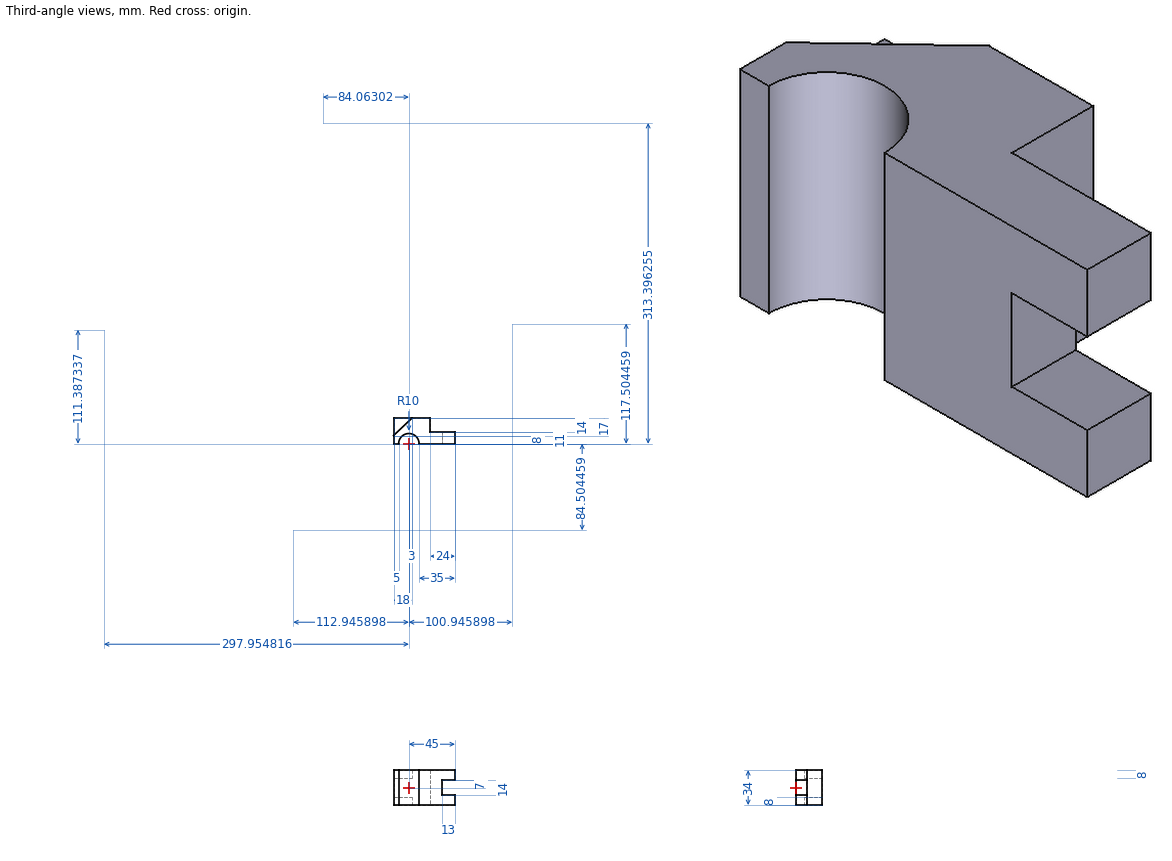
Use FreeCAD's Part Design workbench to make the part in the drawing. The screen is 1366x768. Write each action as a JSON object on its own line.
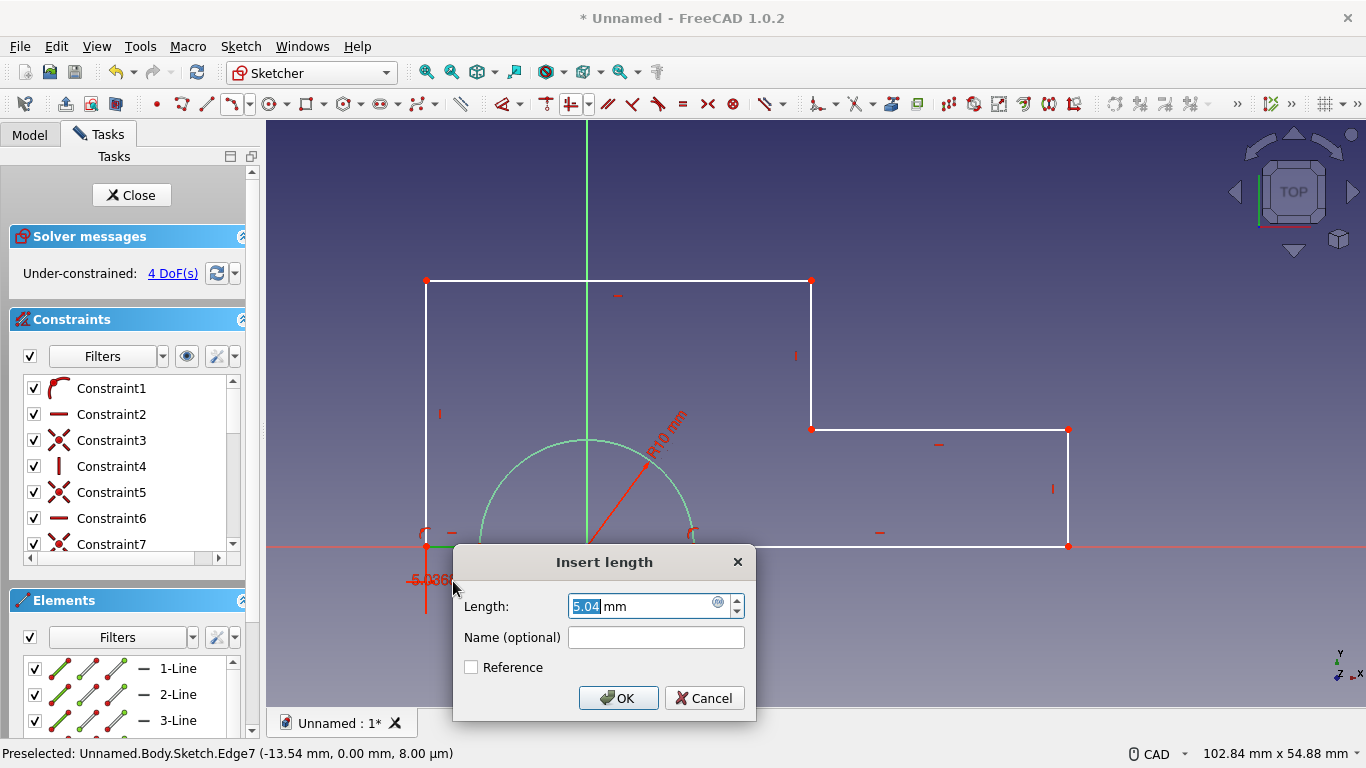
{"action": "type", "text": "5"}
{"action": "key", "text": "Return"}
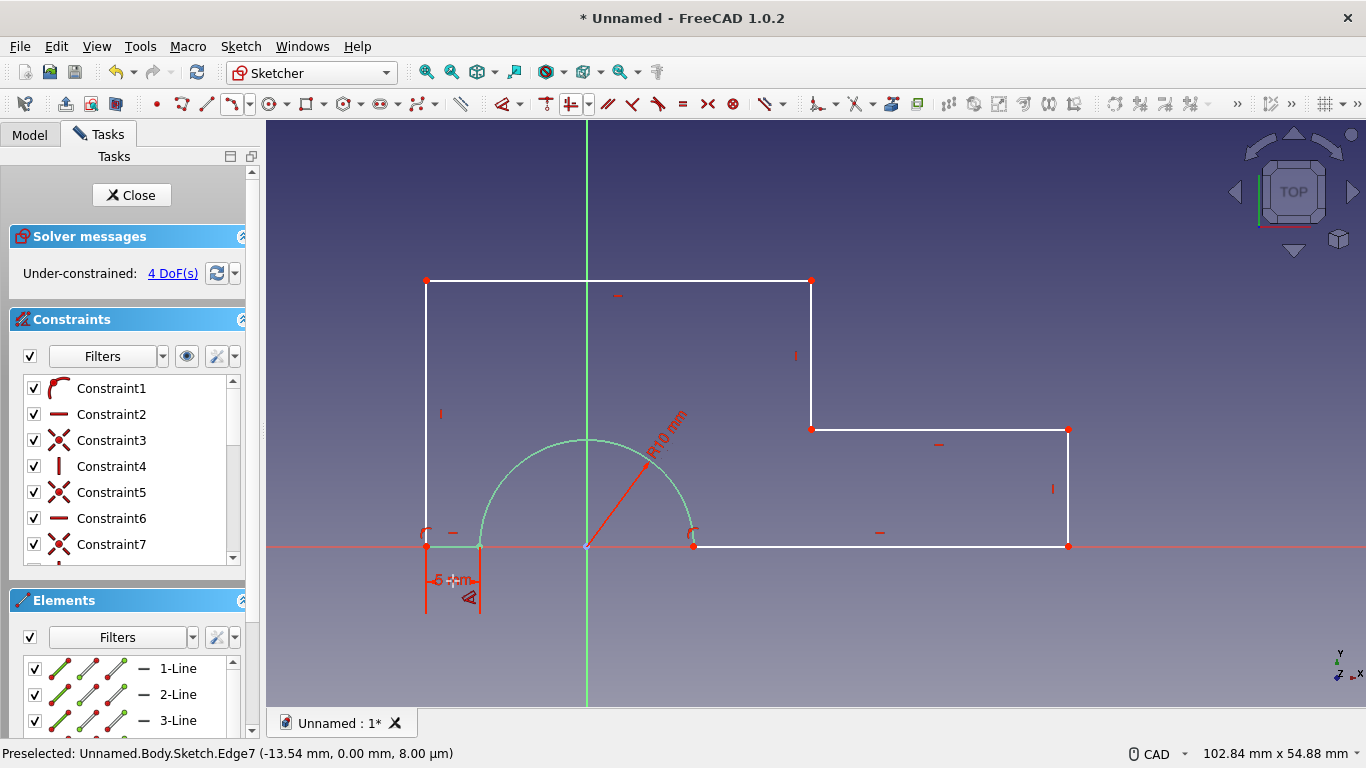
{"action": "left_click", "coordinate": [806, 547]}
{"action": "left_click", "coordinate": [881, 581]}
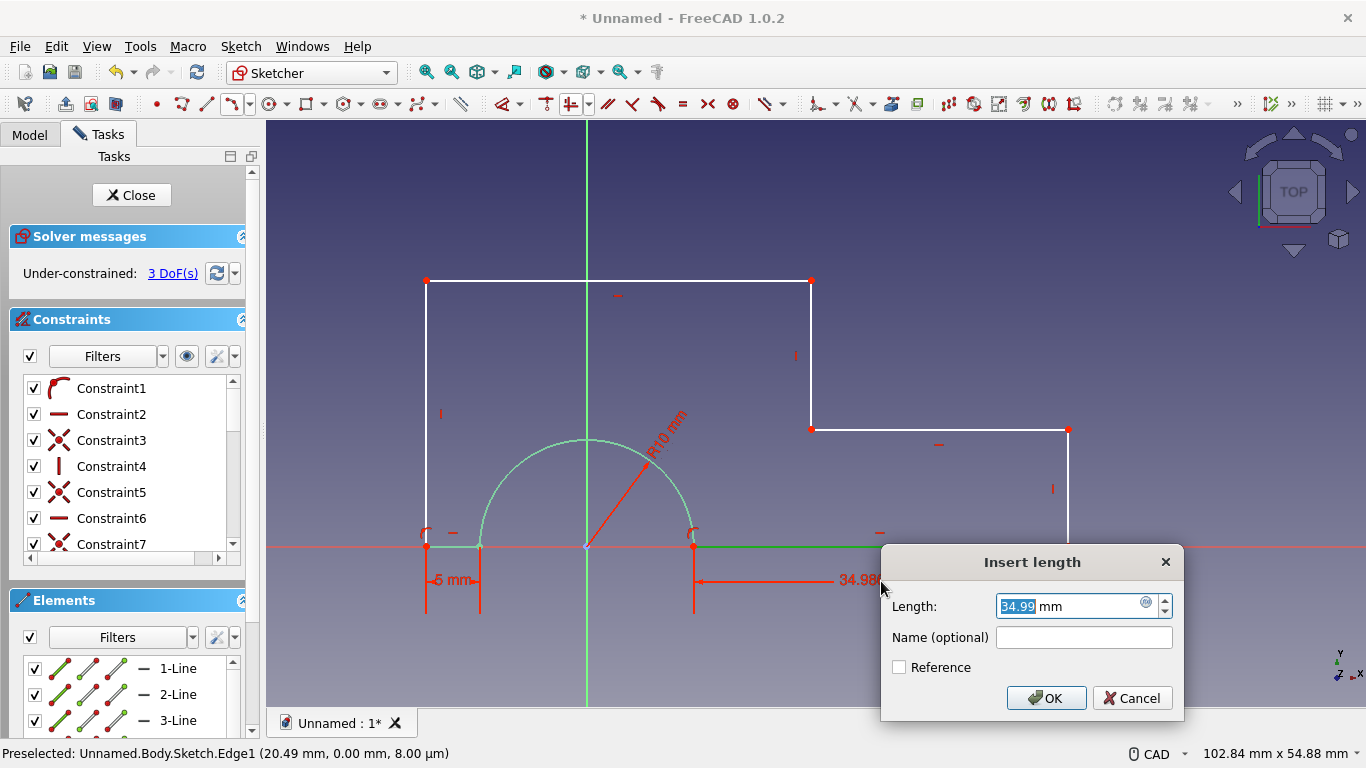
{"action": "type", "text": "35"}
{"action": "key", "text": "Return"}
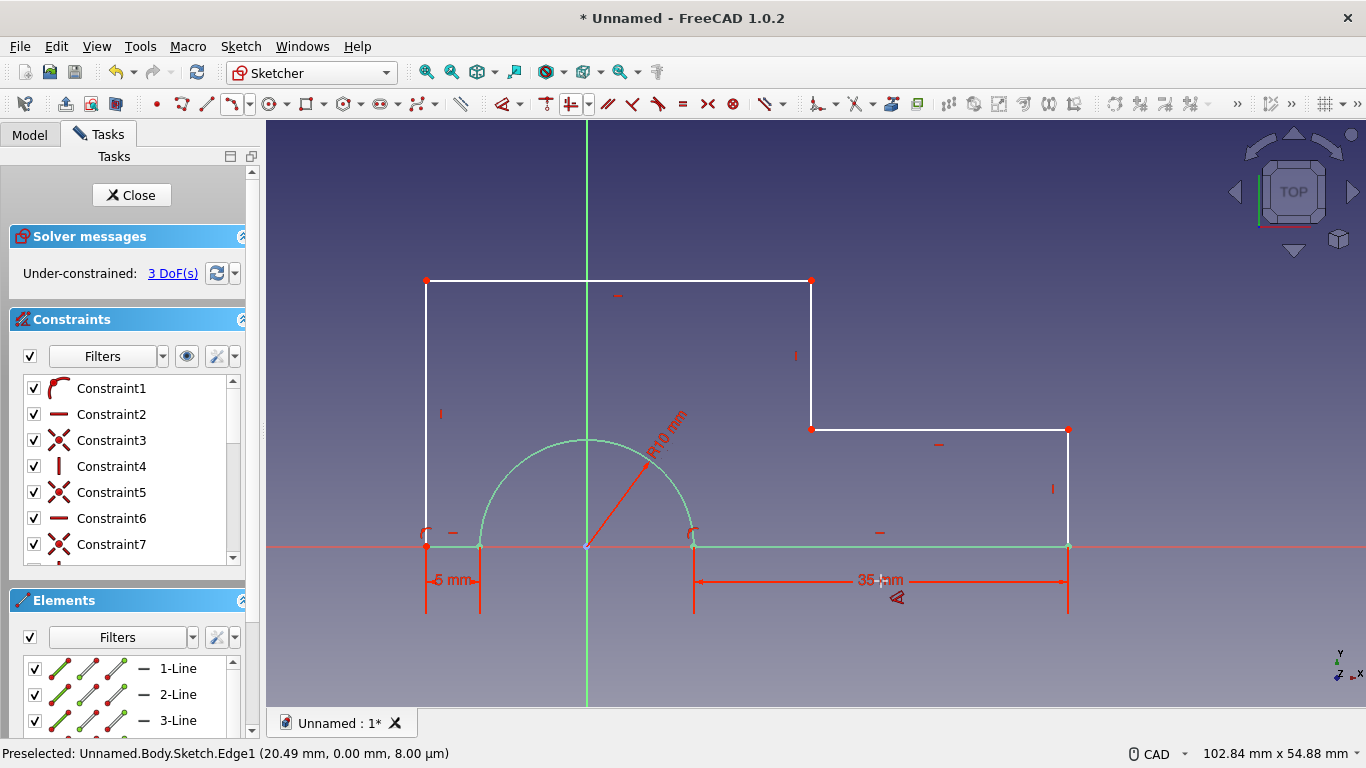
{"action": "left_click", "coordinate": [1068, 512]}
{"action": "left_click", "coordinate": [1102, 488]}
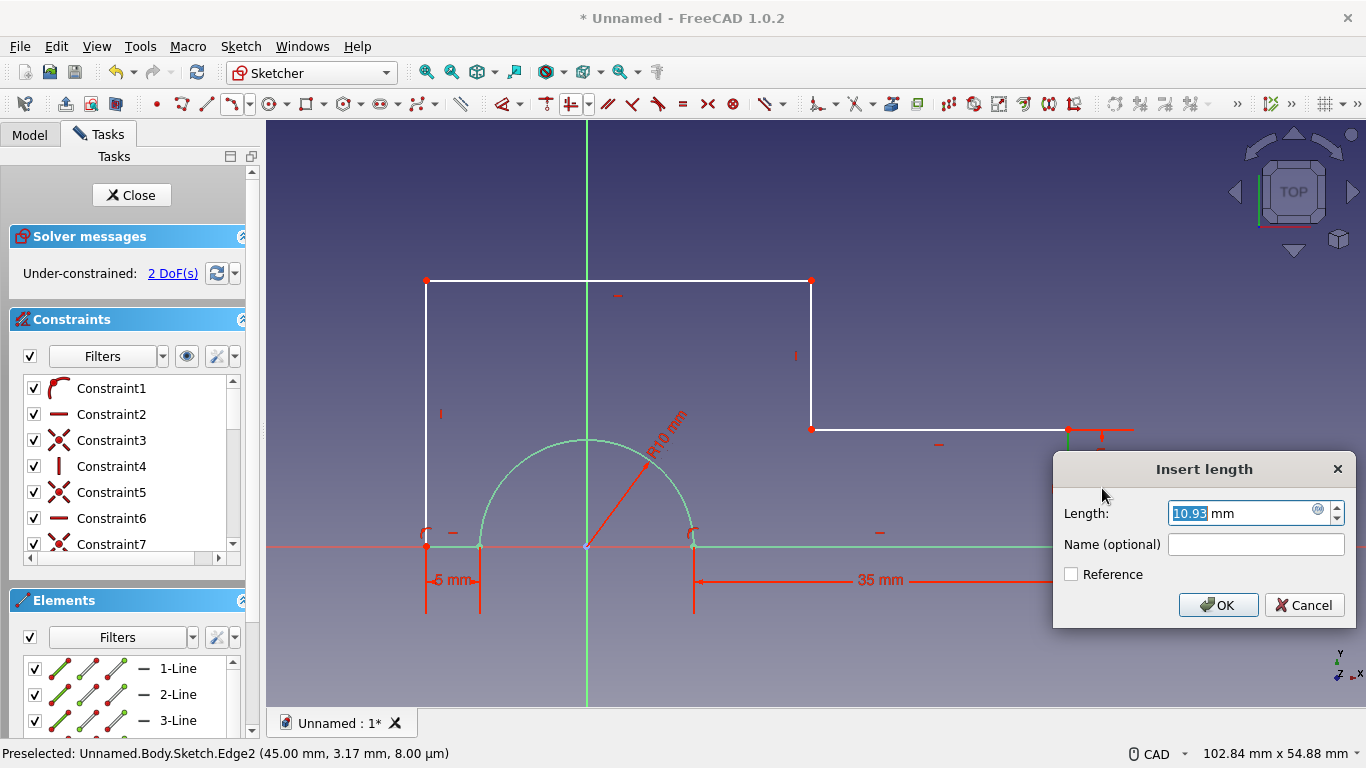
{"action": "type", "text": "11"}
{"action": "key", "text": "Return"}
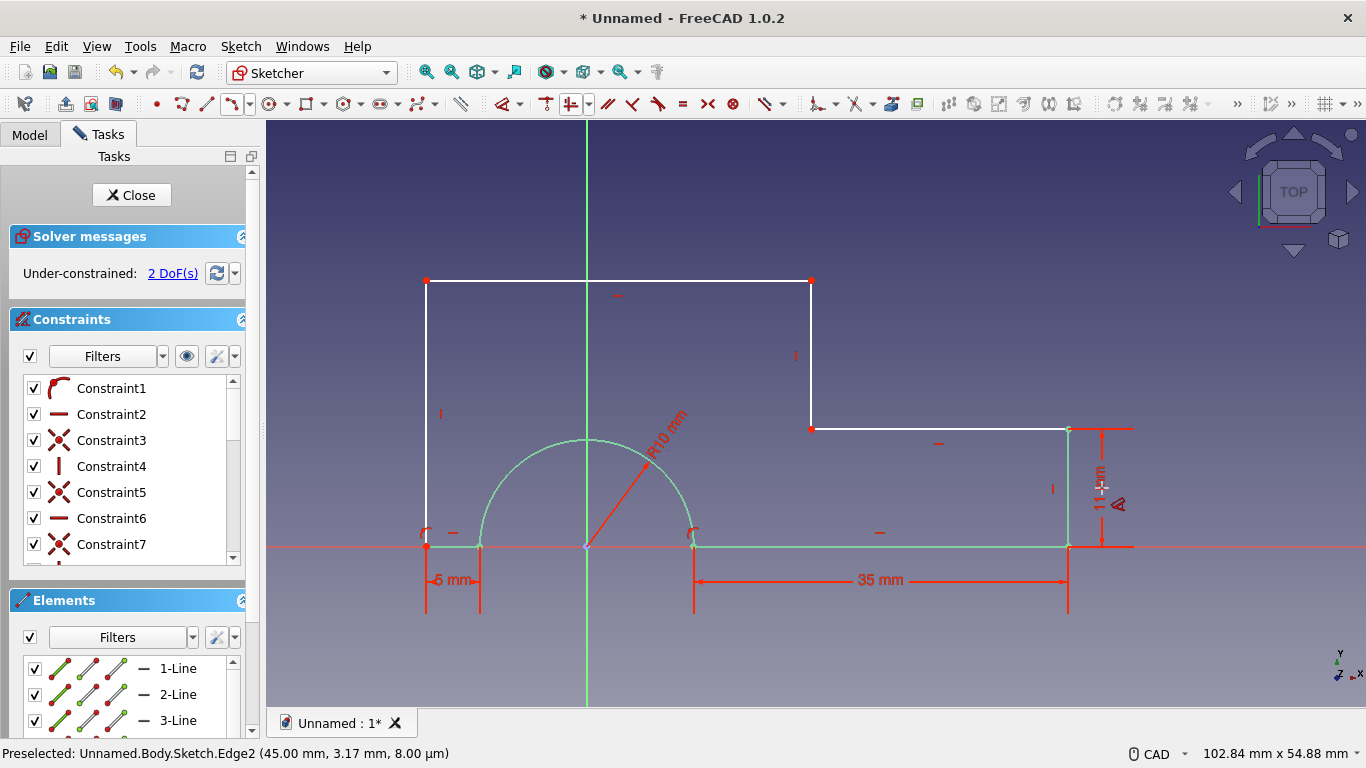
{"action": "left_click", "coordinate": [991, 429]}
{"action": "left_click", "coordinate": [940, 463]}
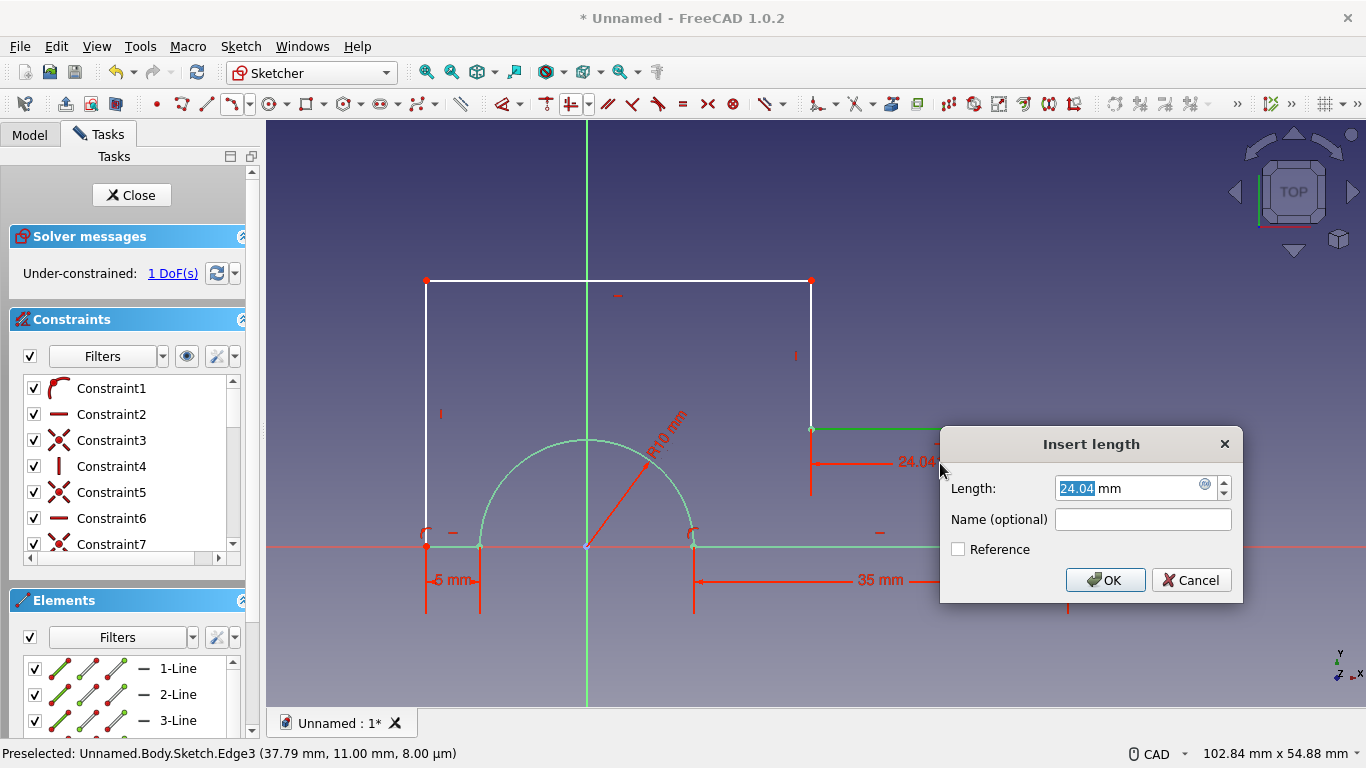
{"action": "type", "text": "24"}
{"action": "key", "text": "Return"}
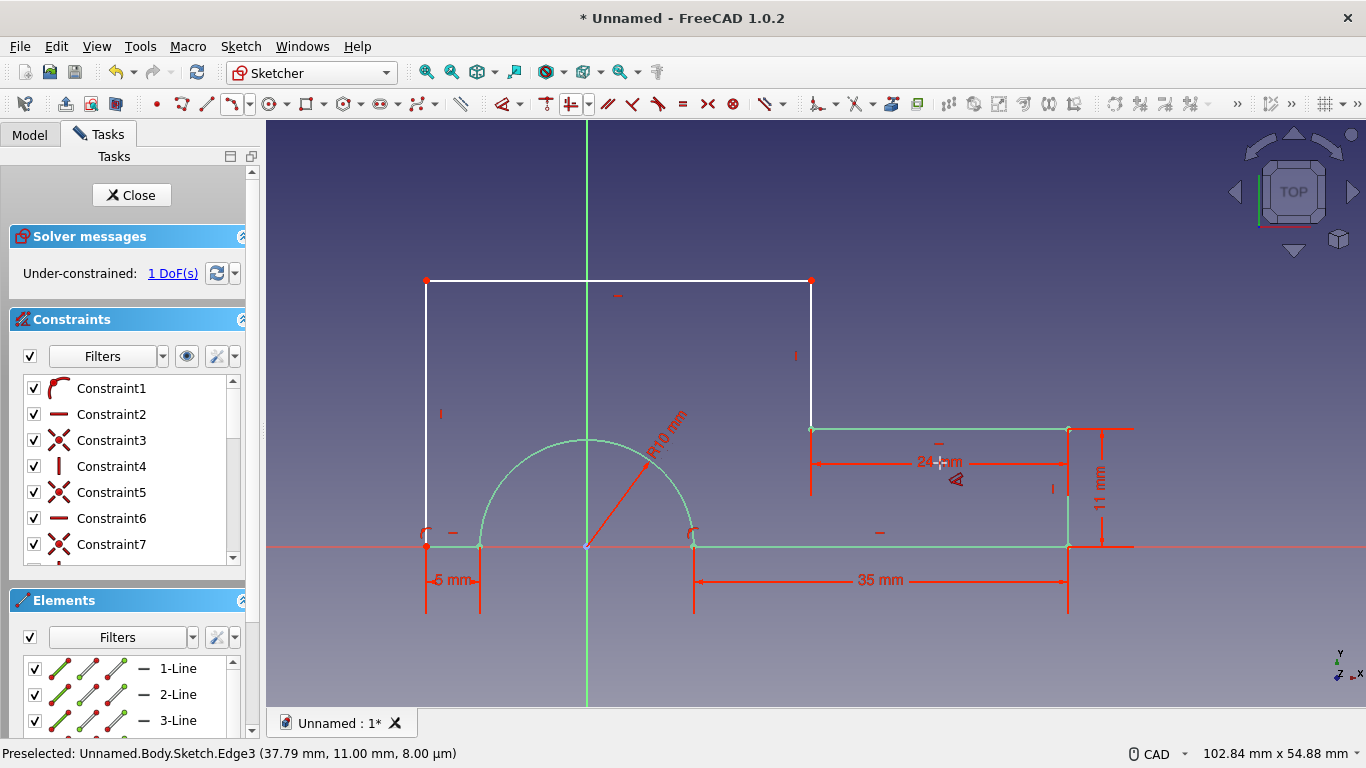
{"action": "left_click", "coordinate": [811, 385]}
{"action": "left_click", "coordinate": [845, 355]}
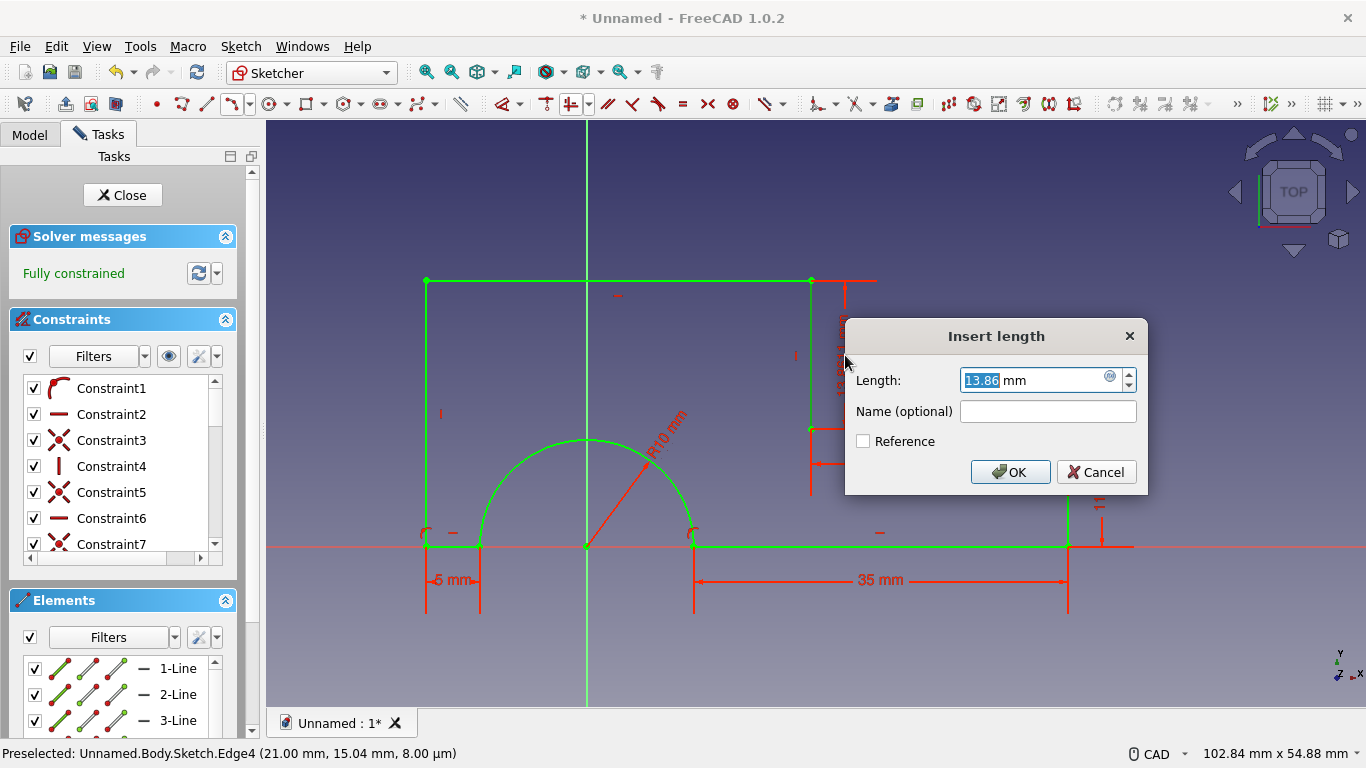
{"action": "type", "text": "14"}
{"action": "key", "text": "Return"}
{"action": "key", "text": "Escape"}